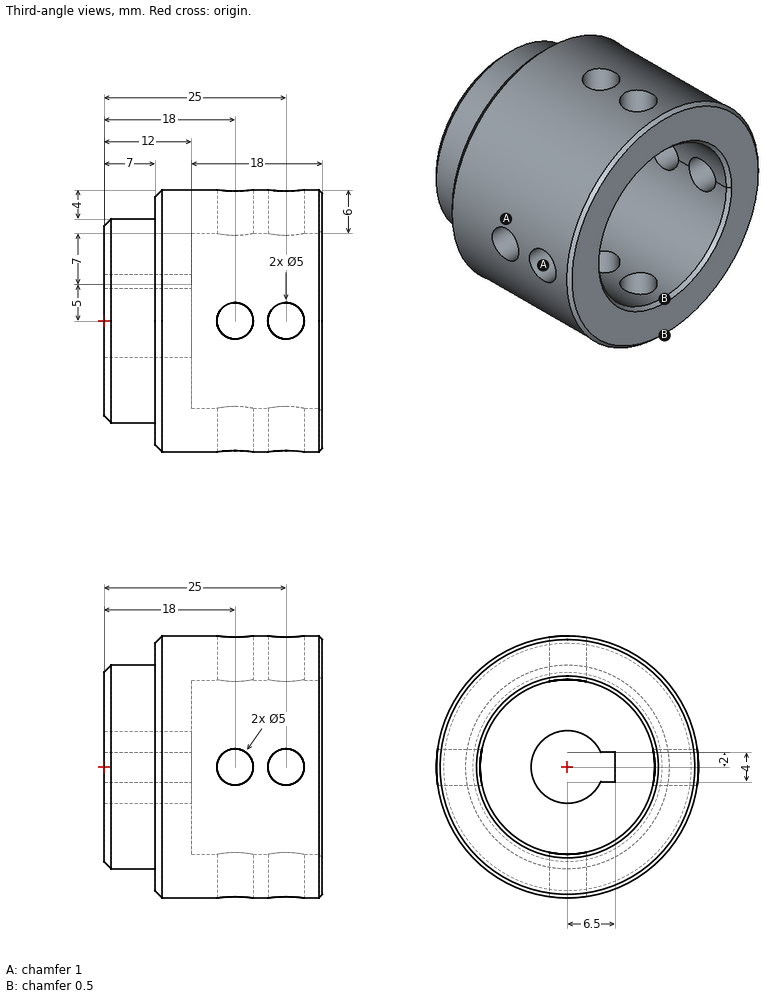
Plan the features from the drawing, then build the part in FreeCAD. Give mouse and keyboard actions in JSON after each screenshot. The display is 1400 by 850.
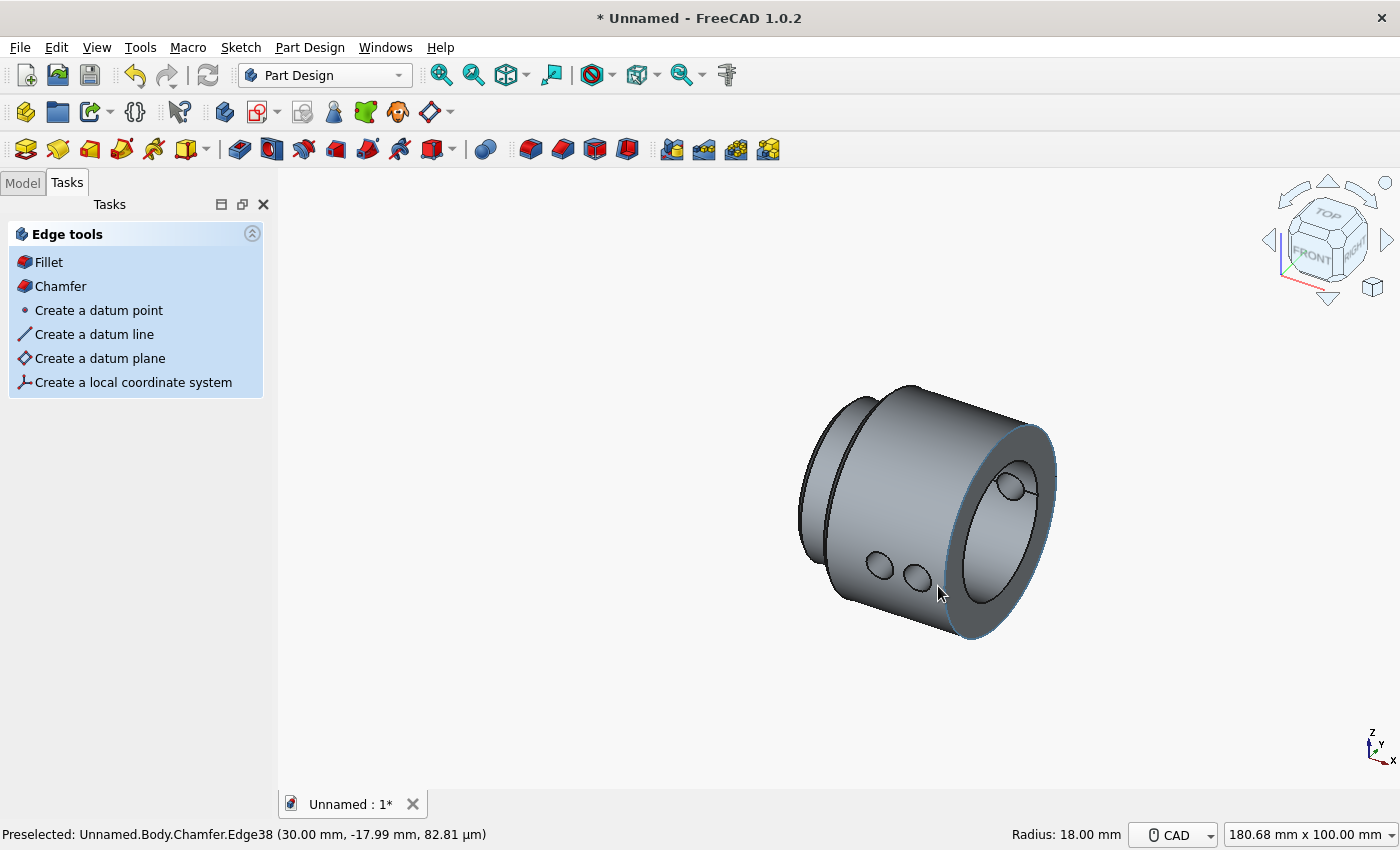
{"action": "left_click", "coordinate": [989, 600], "text": "ctrl"}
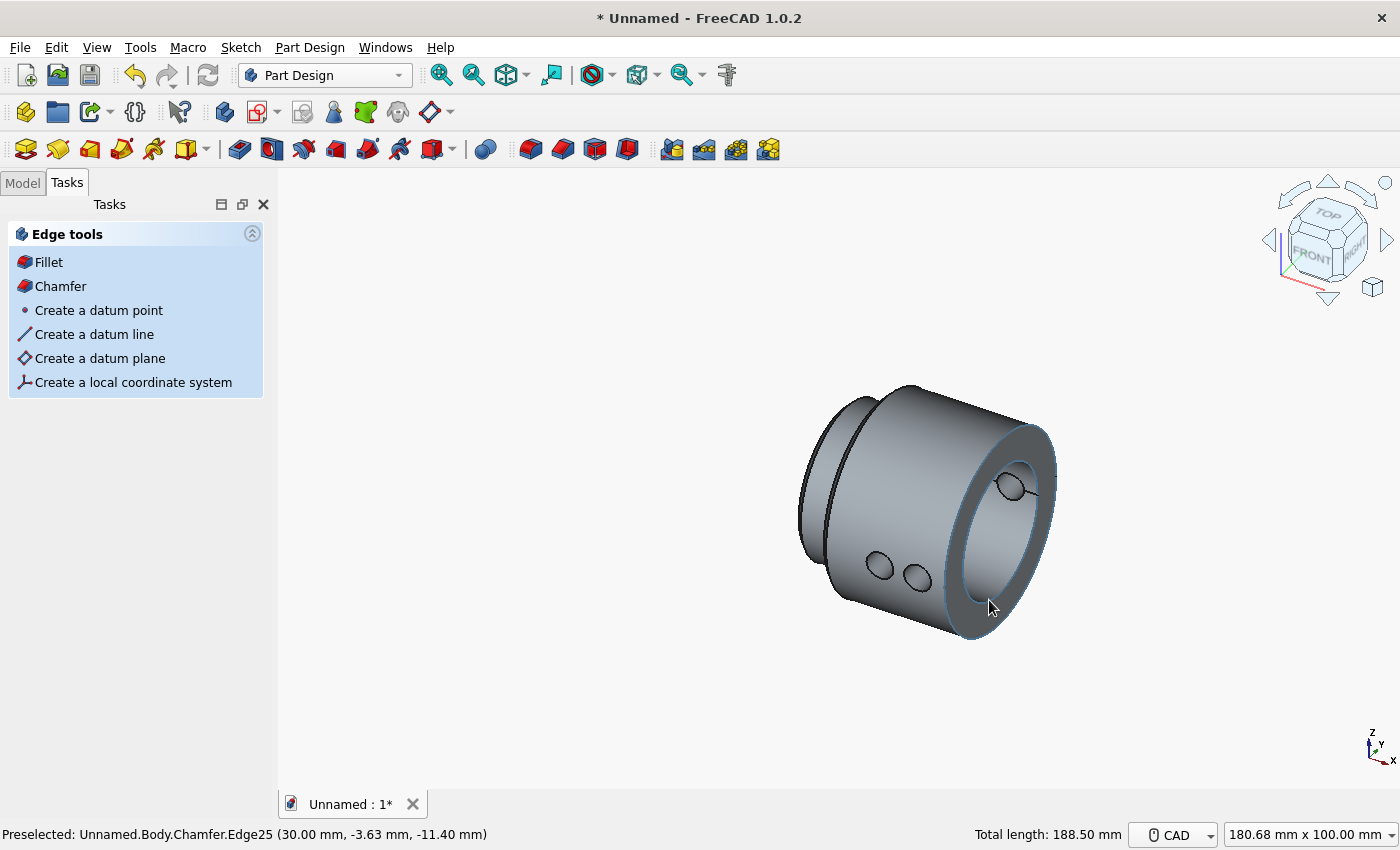
{"action": "left_click", "coordinate": [564, 150]}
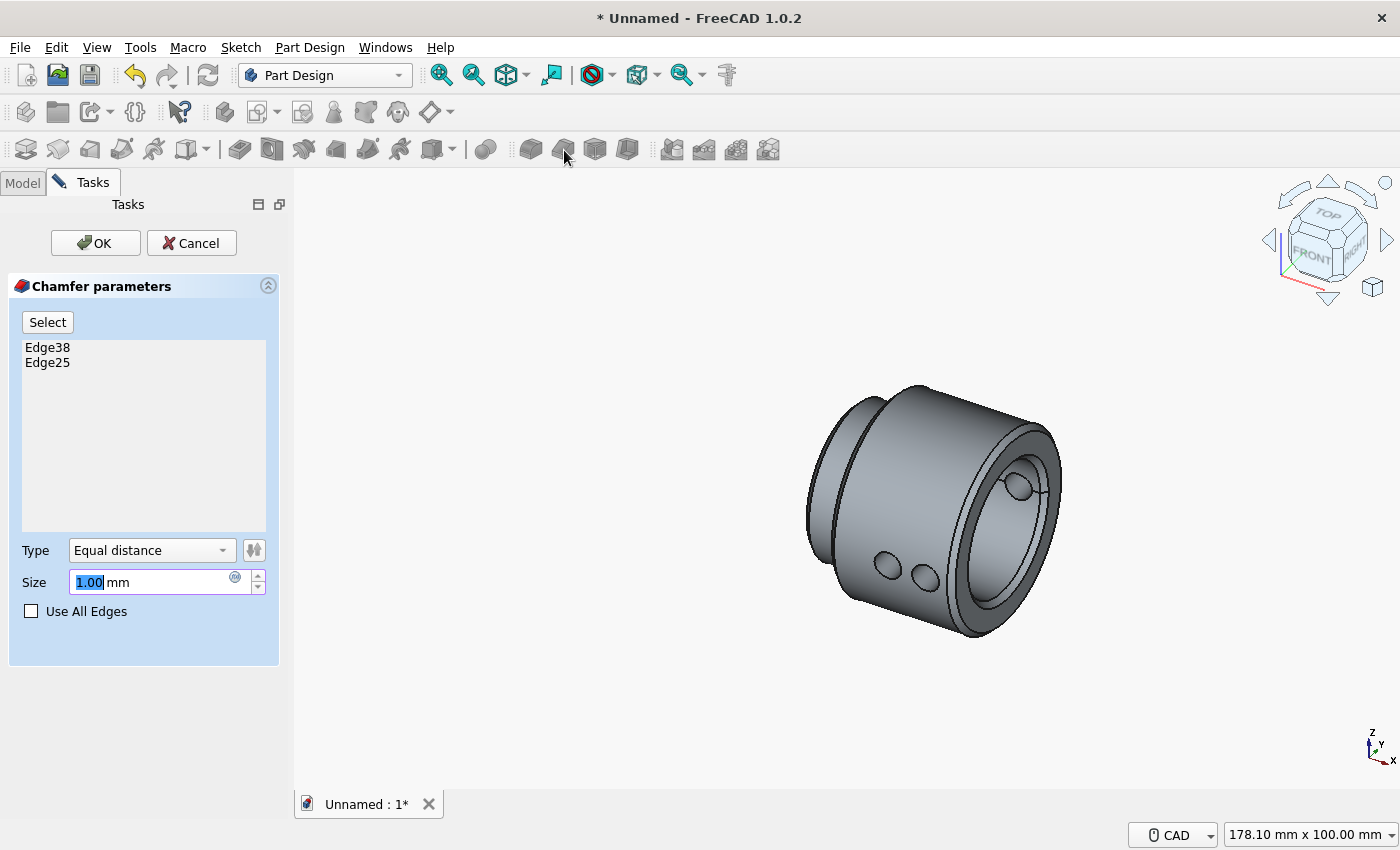
{"action": "type", "text": "0.5"}
{"action": "key", "text": "Tab"}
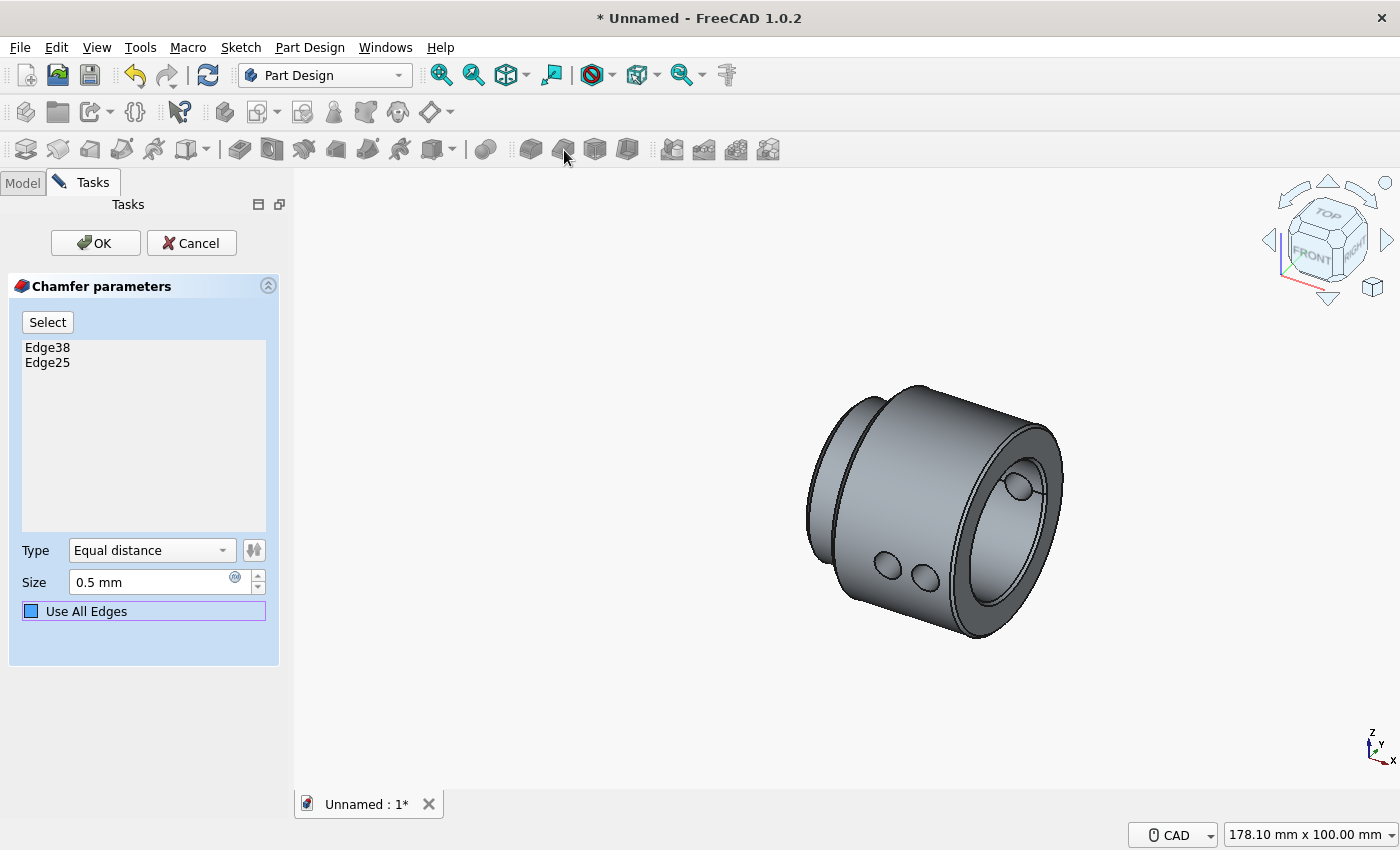
{"action": "left_click", "coordinate": [96, 243]}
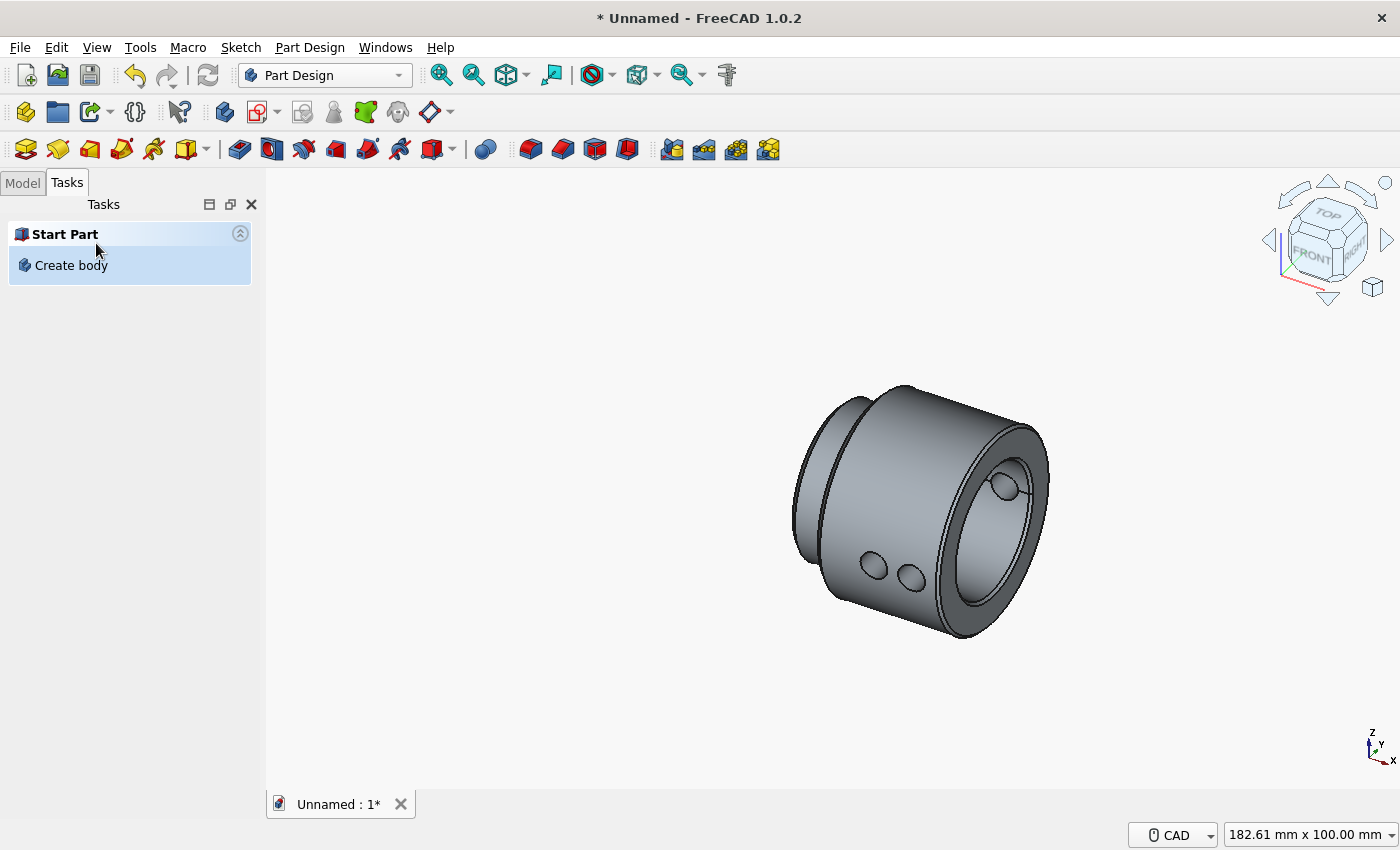
{"action": "left_click", "coordinate": [258, 112]}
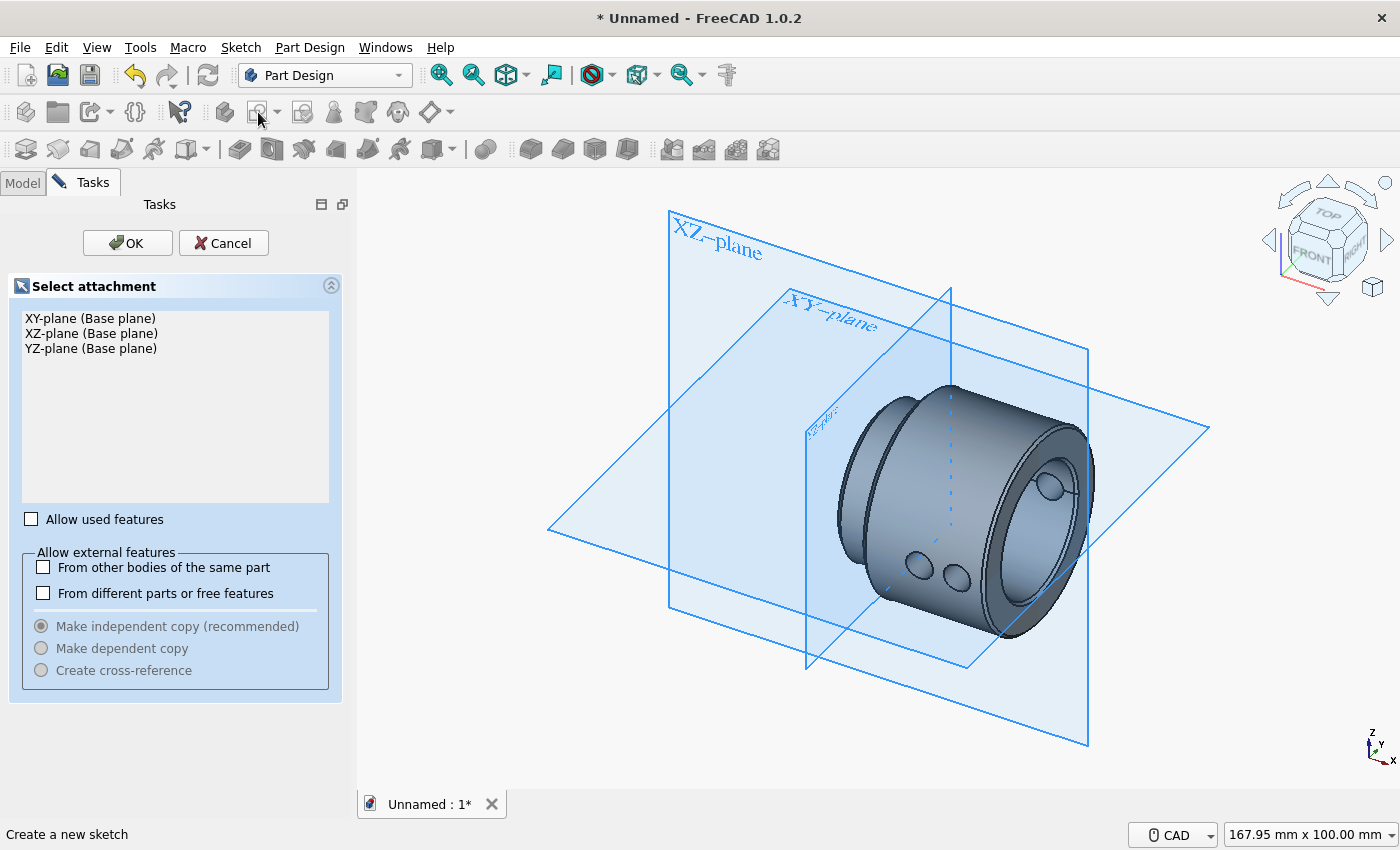
{"action": "left_click", "coordinate": [82, 318]}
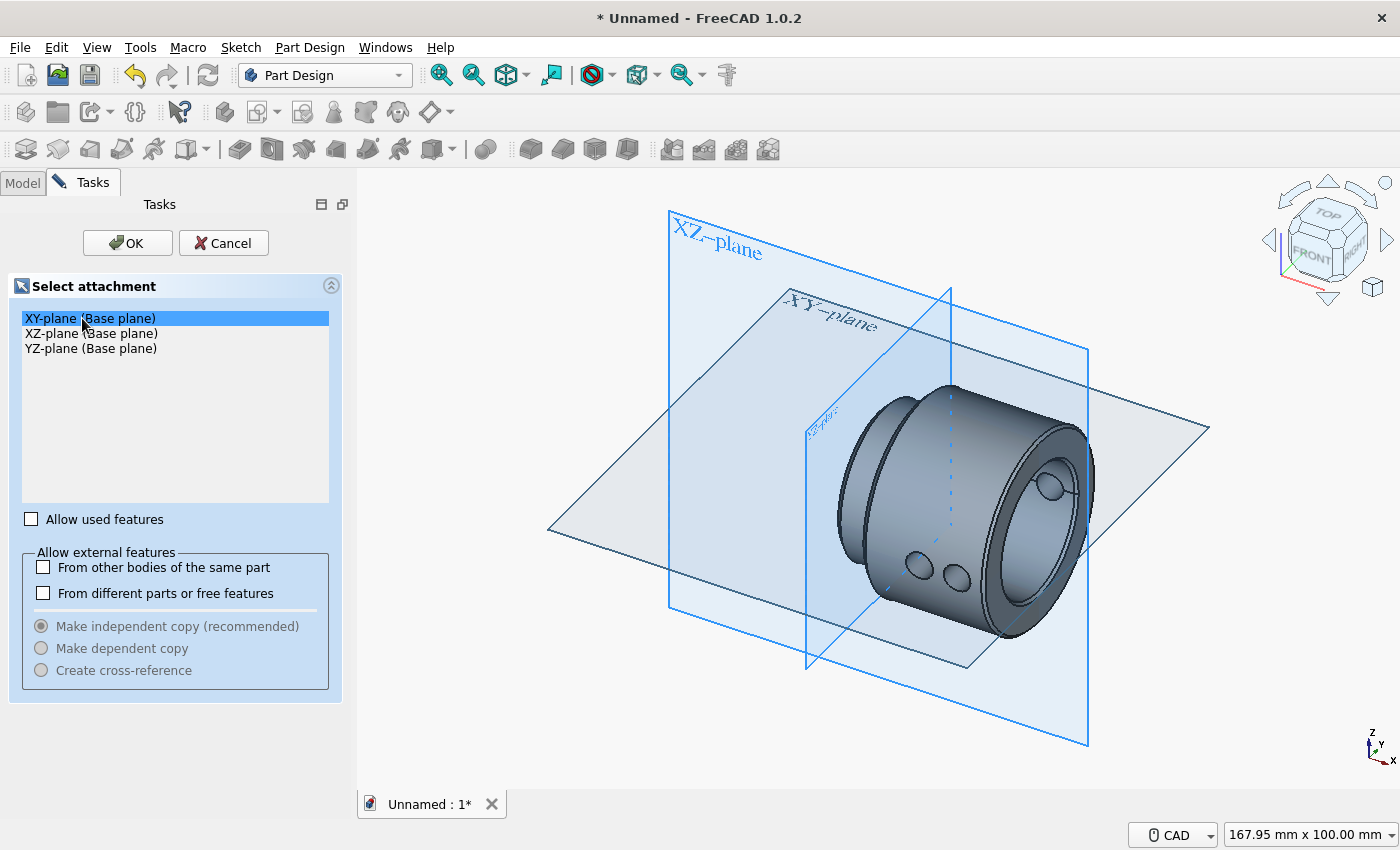
{"action": "left_click", "coordinate": [128, 243]}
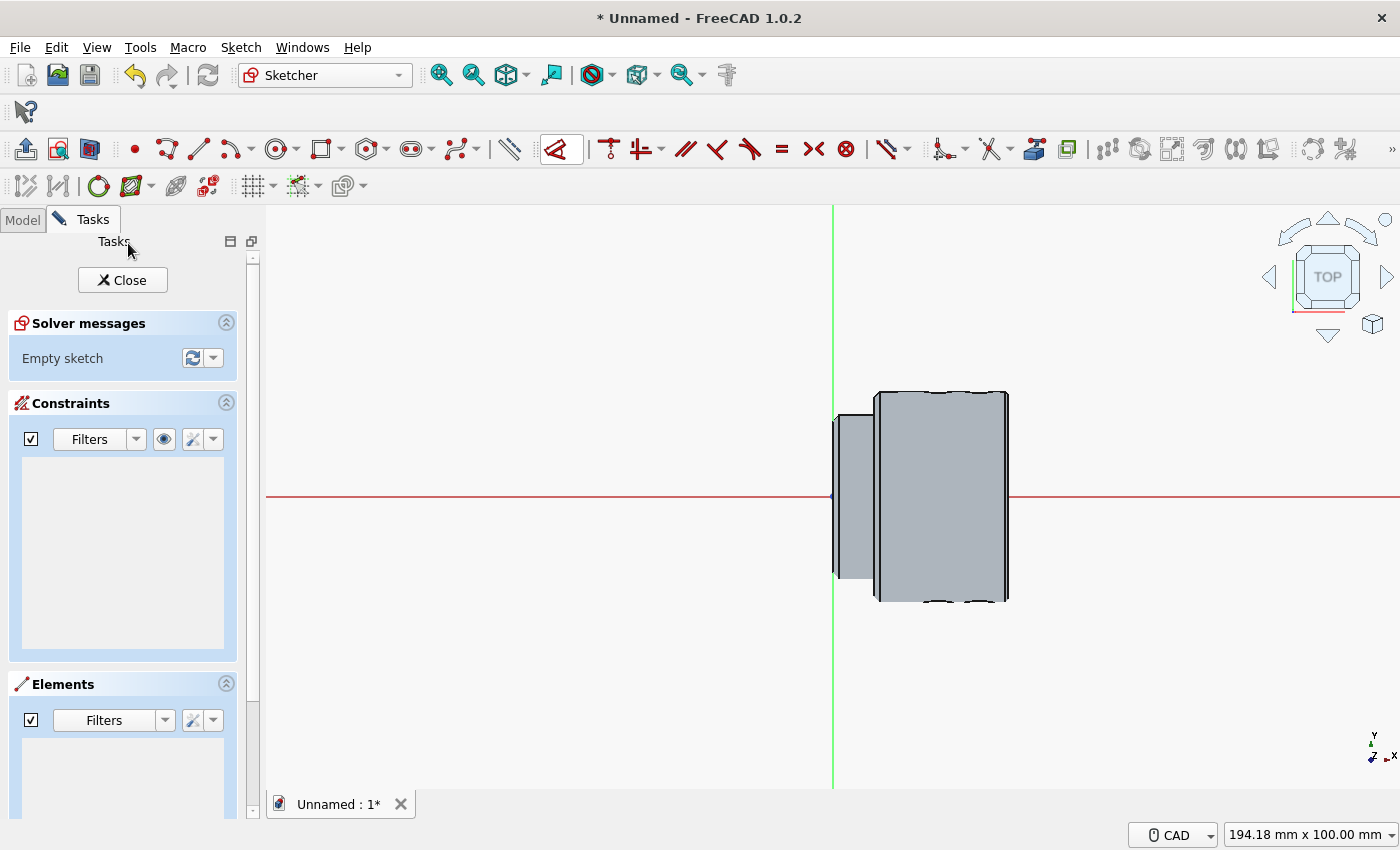
{"action": "left_click", "coordinate": [90, 150]}